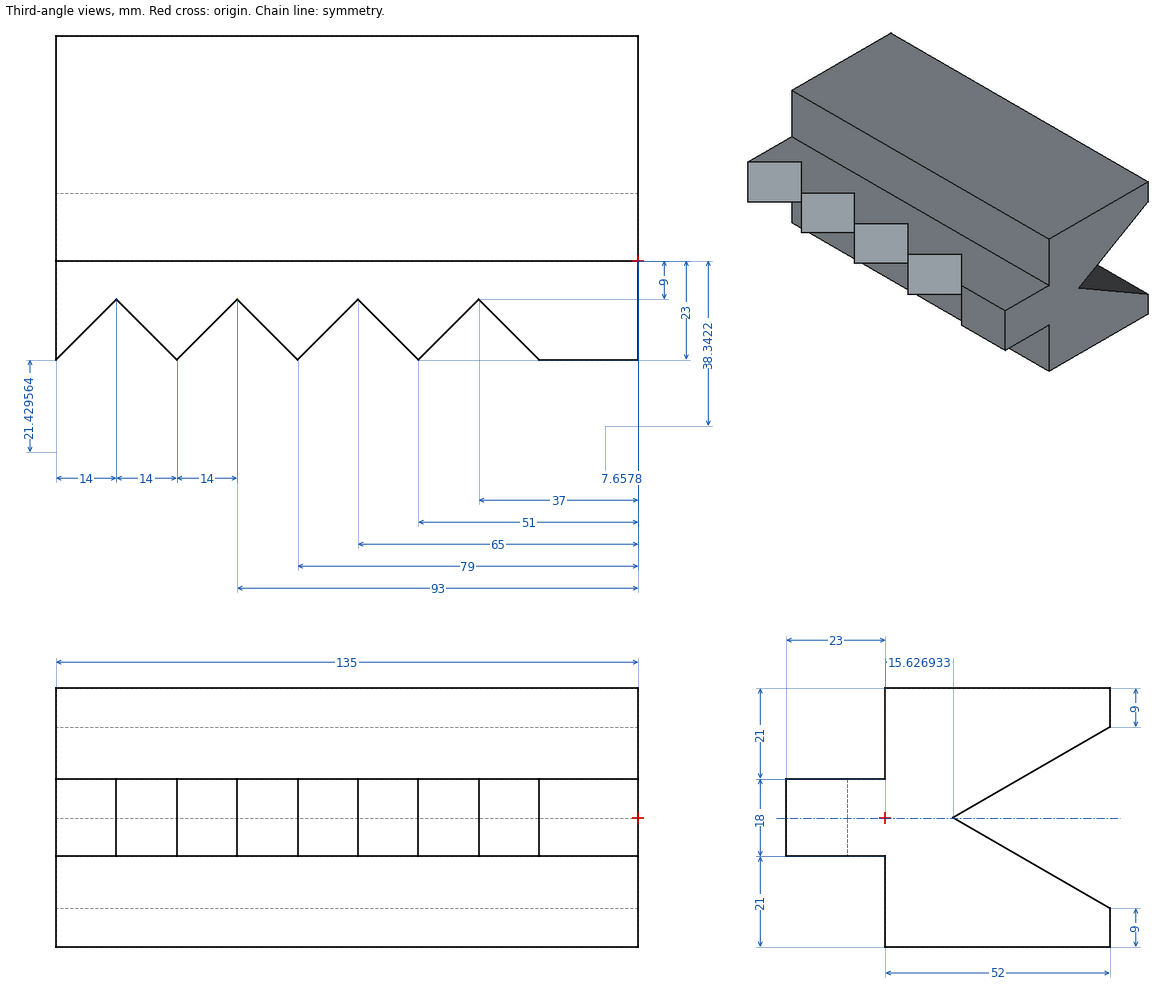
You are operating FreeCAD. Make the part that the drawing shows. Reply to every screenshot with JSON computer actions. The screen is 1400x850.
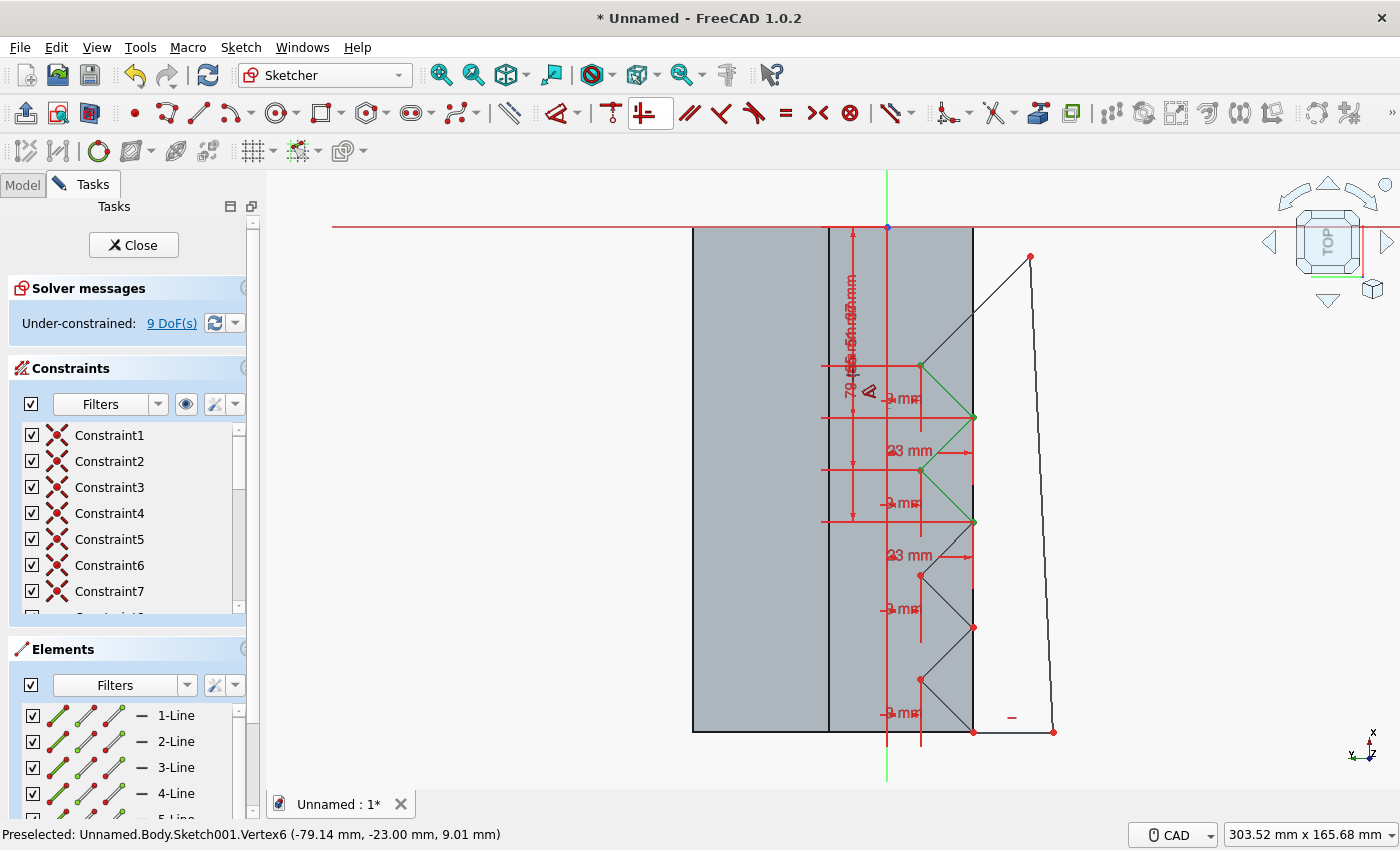
{"action": "left_click", "coordinate": [921, 576]}
{"action": "left_click", "coordinate": [853, 482]}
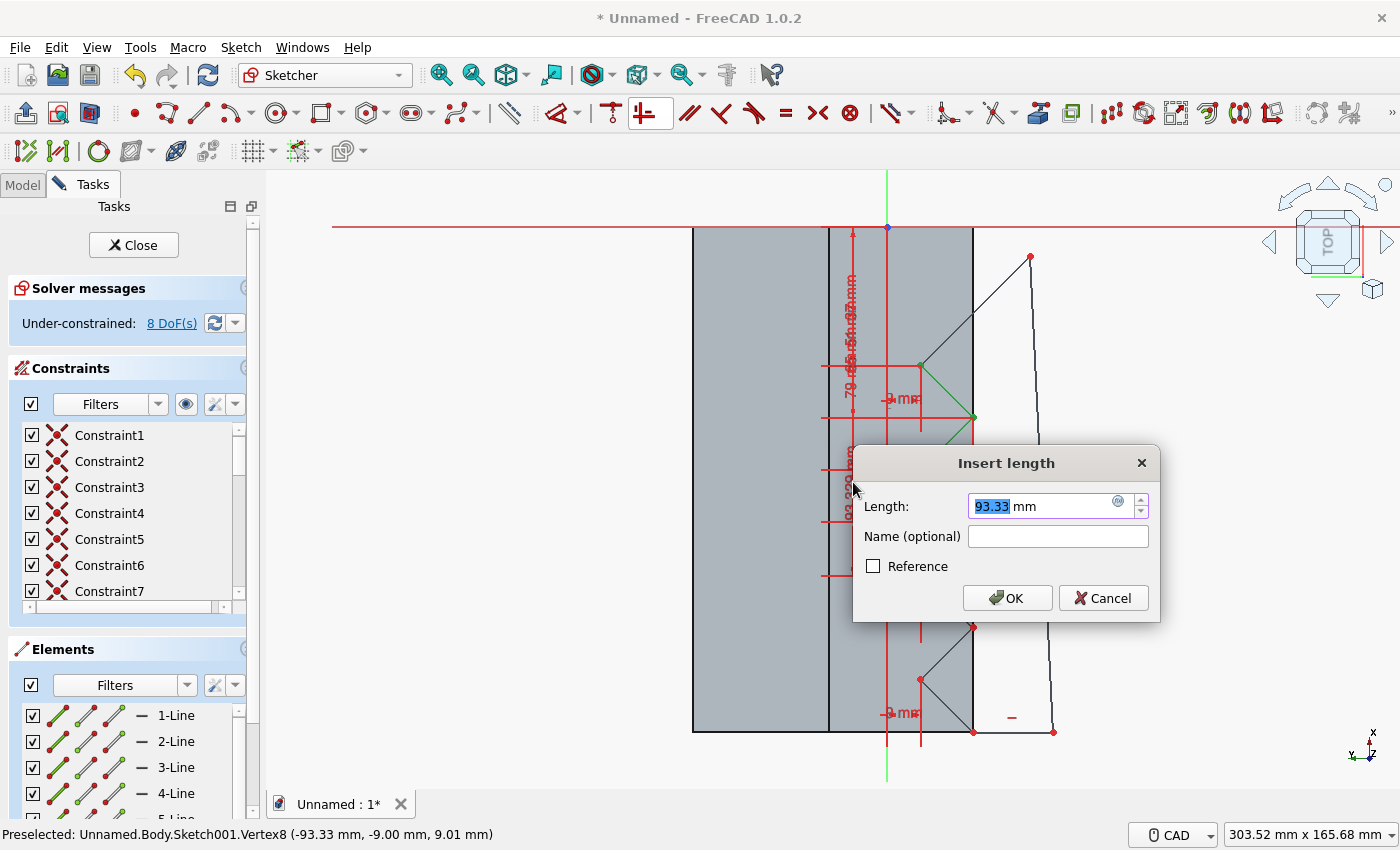
{"action": "type", "text": "93"}
{"action": "key", "text": "Return"}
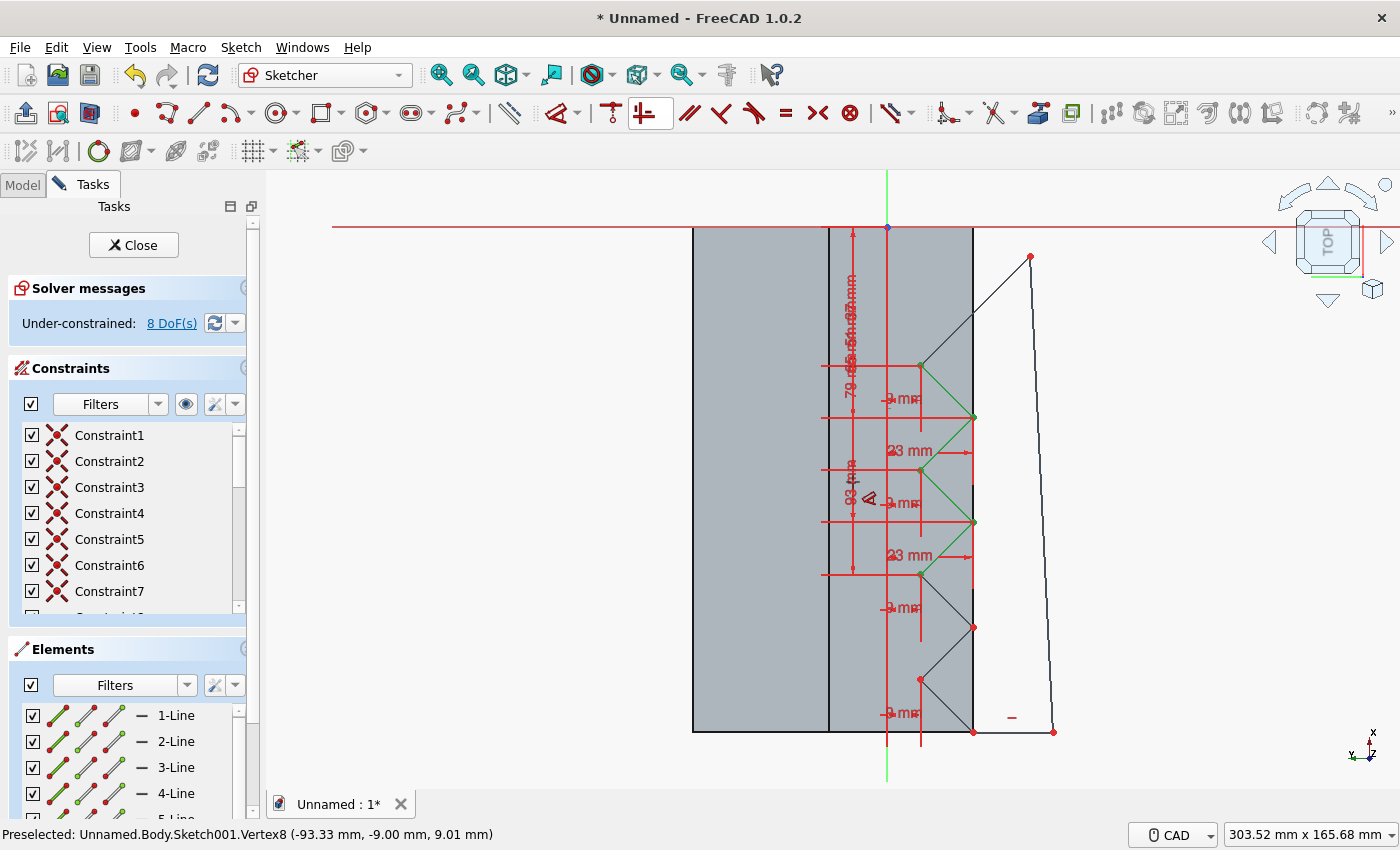
{"action": "left_click", "coordinate": [973, 628]}
{"action": "left_click", "coordinate": [910, 662]}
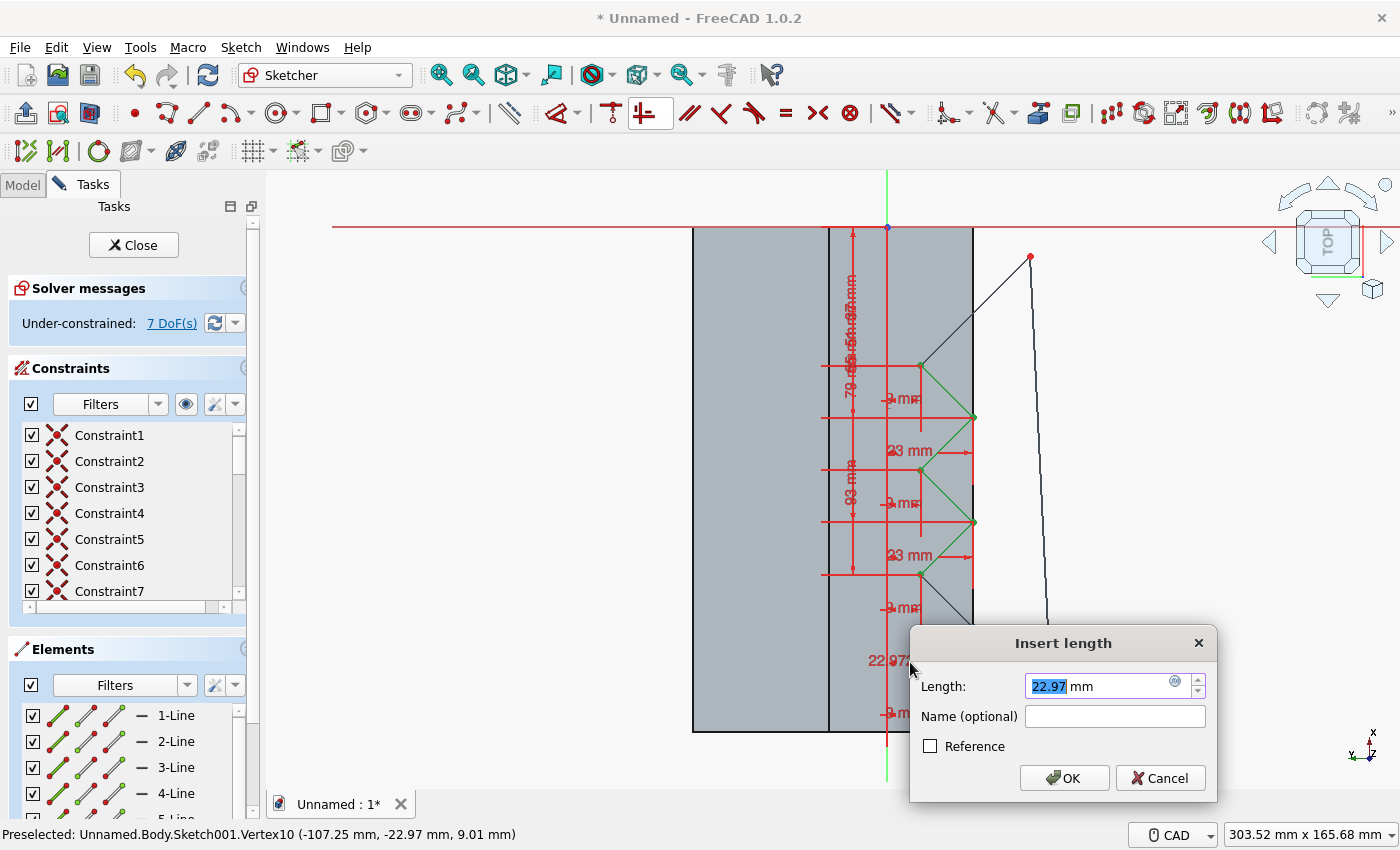
{"action": "type", "text": "23"}
{"action": "key", "text": "Return"}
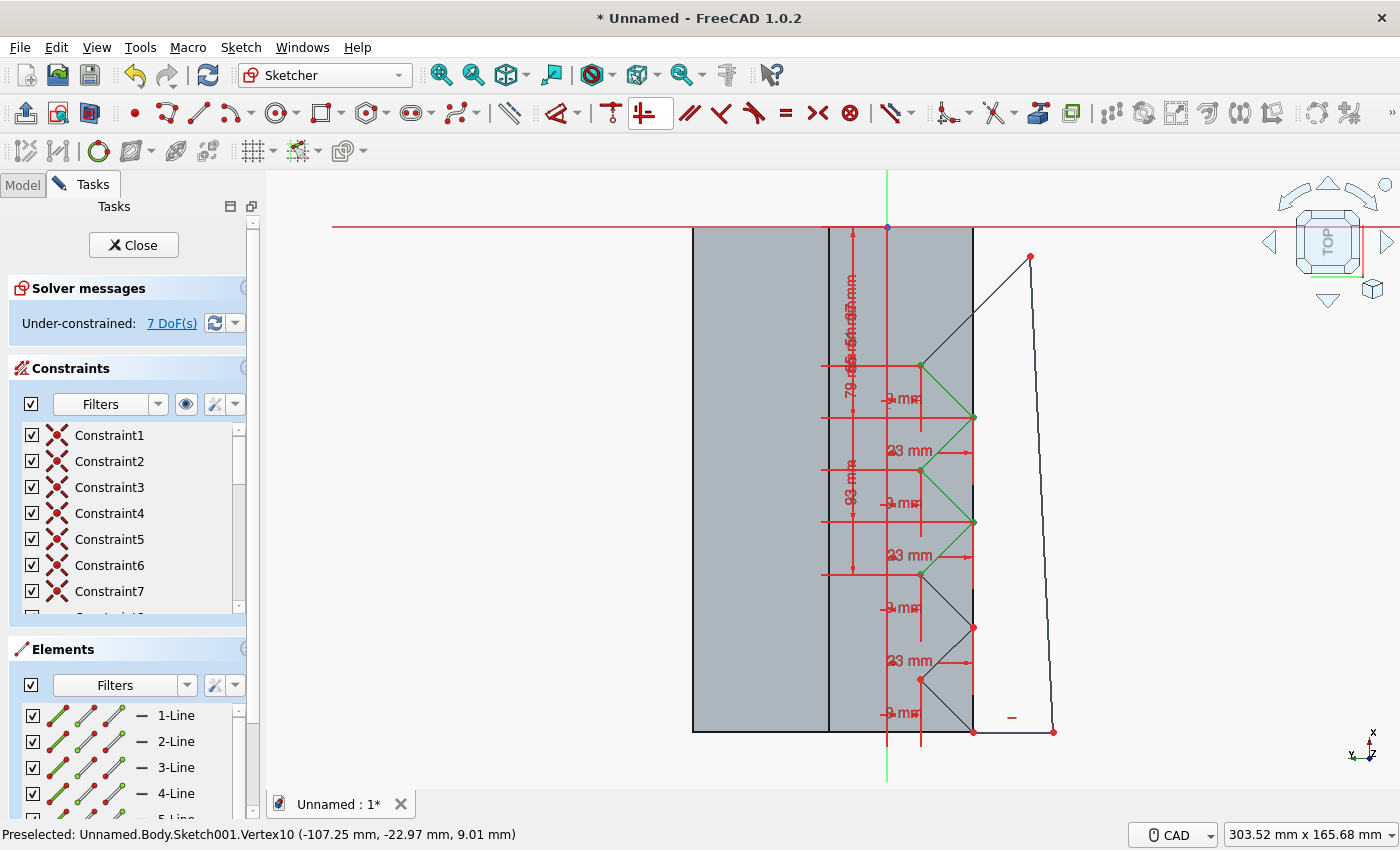
{"action": "left_click", "coordinate": [973, 733]}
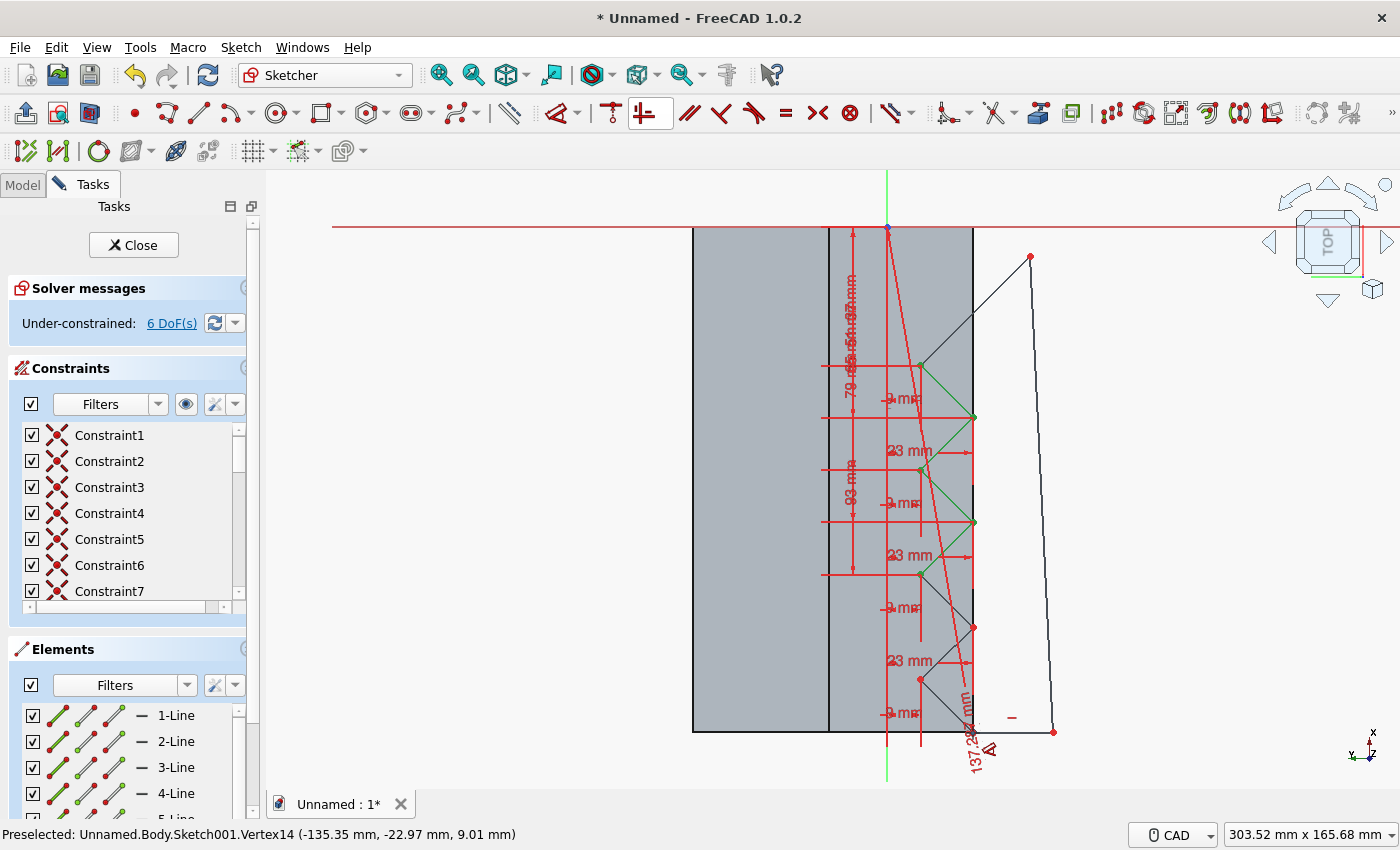
{"action": "key", "text": "Escape"}
{"action": "key", "text": "Escape"}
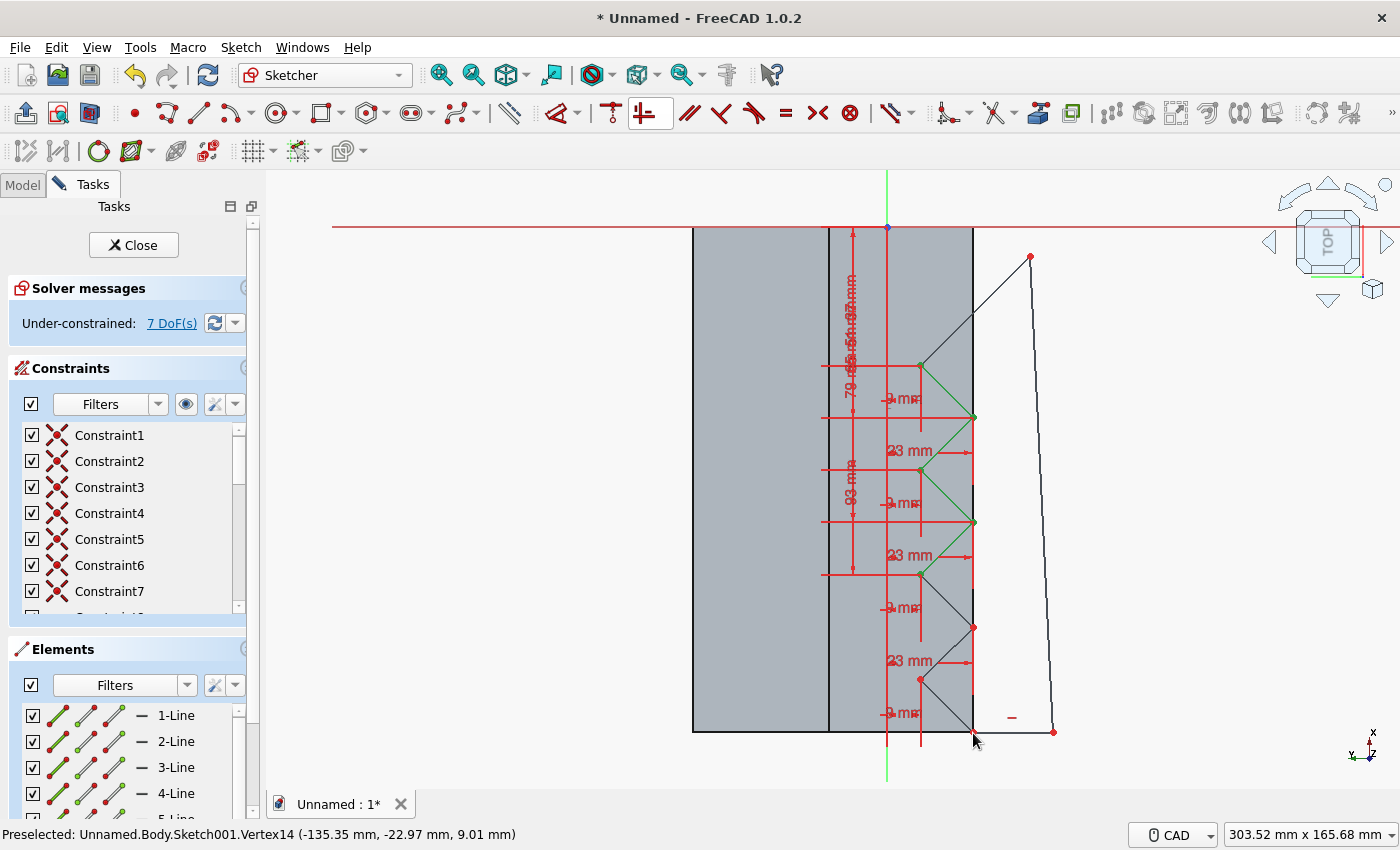
{"action": "left_click", "coordinate": [973, 733]}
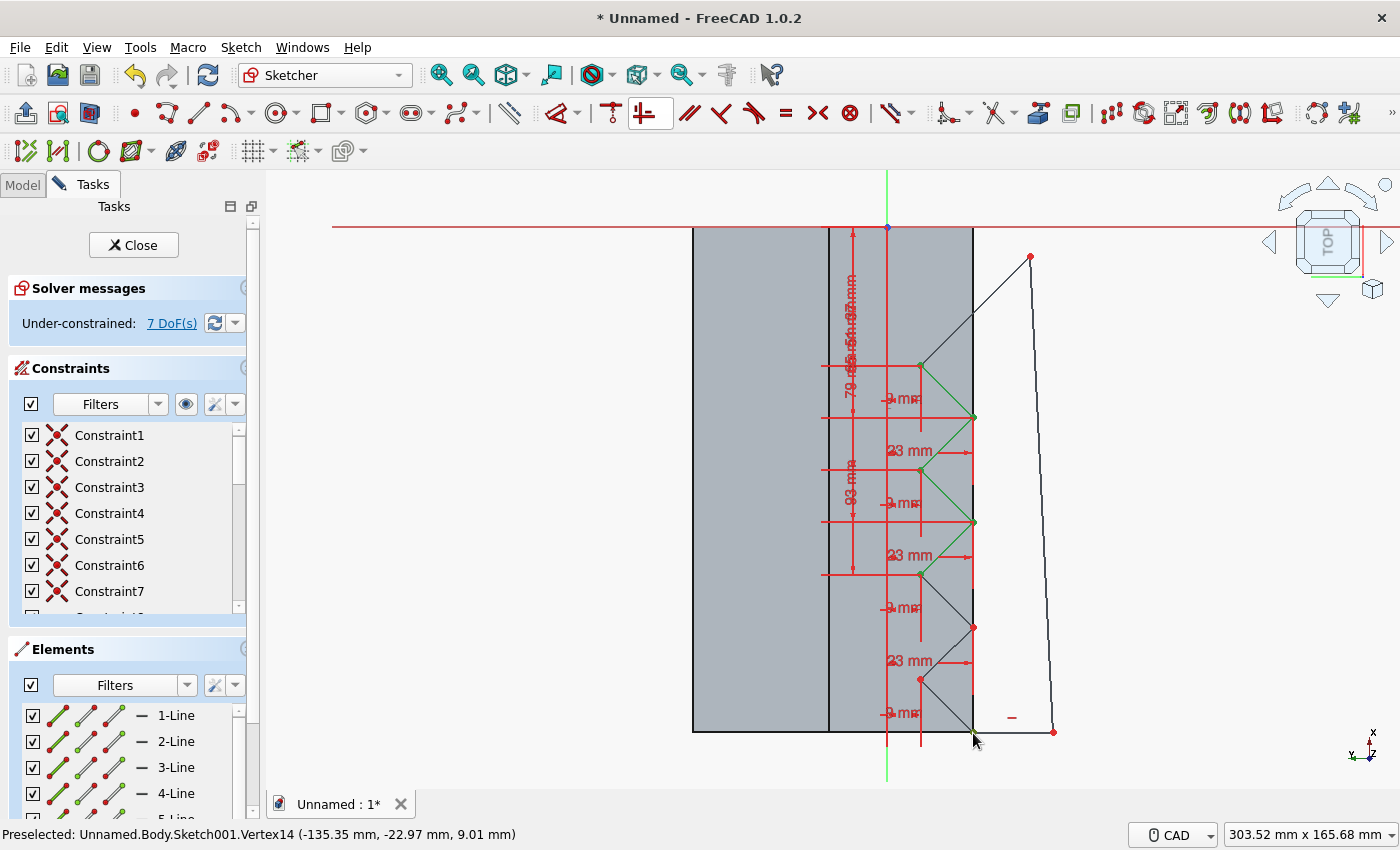
{"action": "key", "text": "l"}